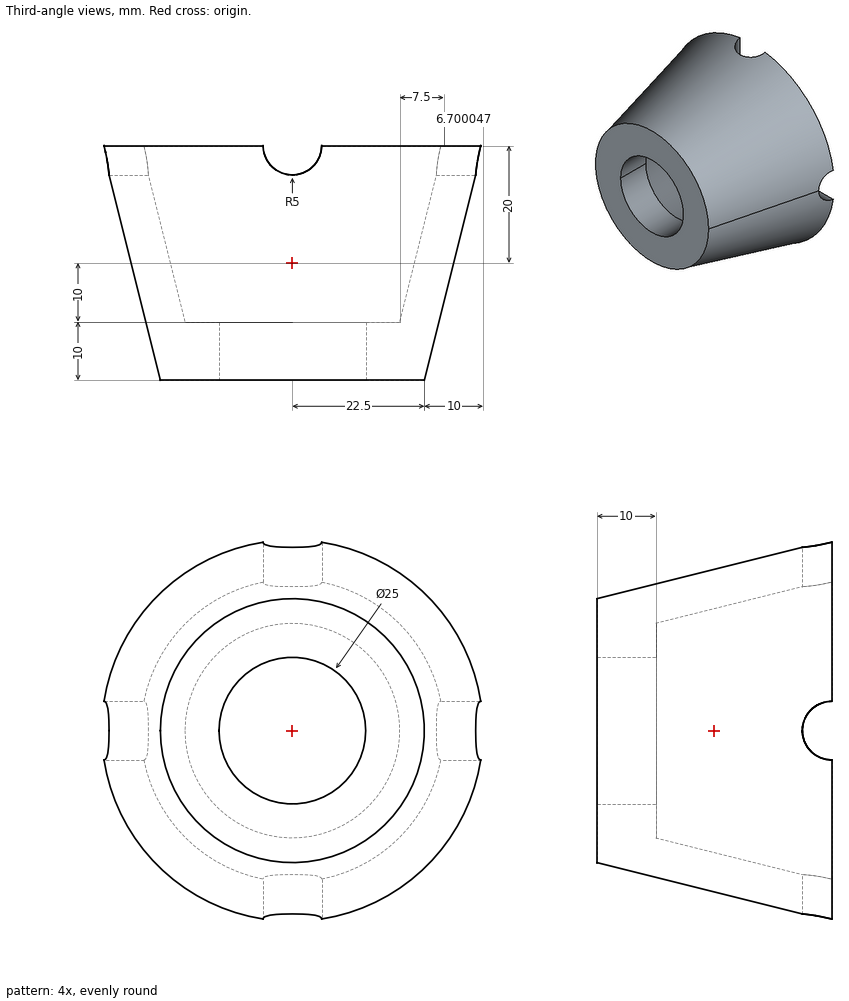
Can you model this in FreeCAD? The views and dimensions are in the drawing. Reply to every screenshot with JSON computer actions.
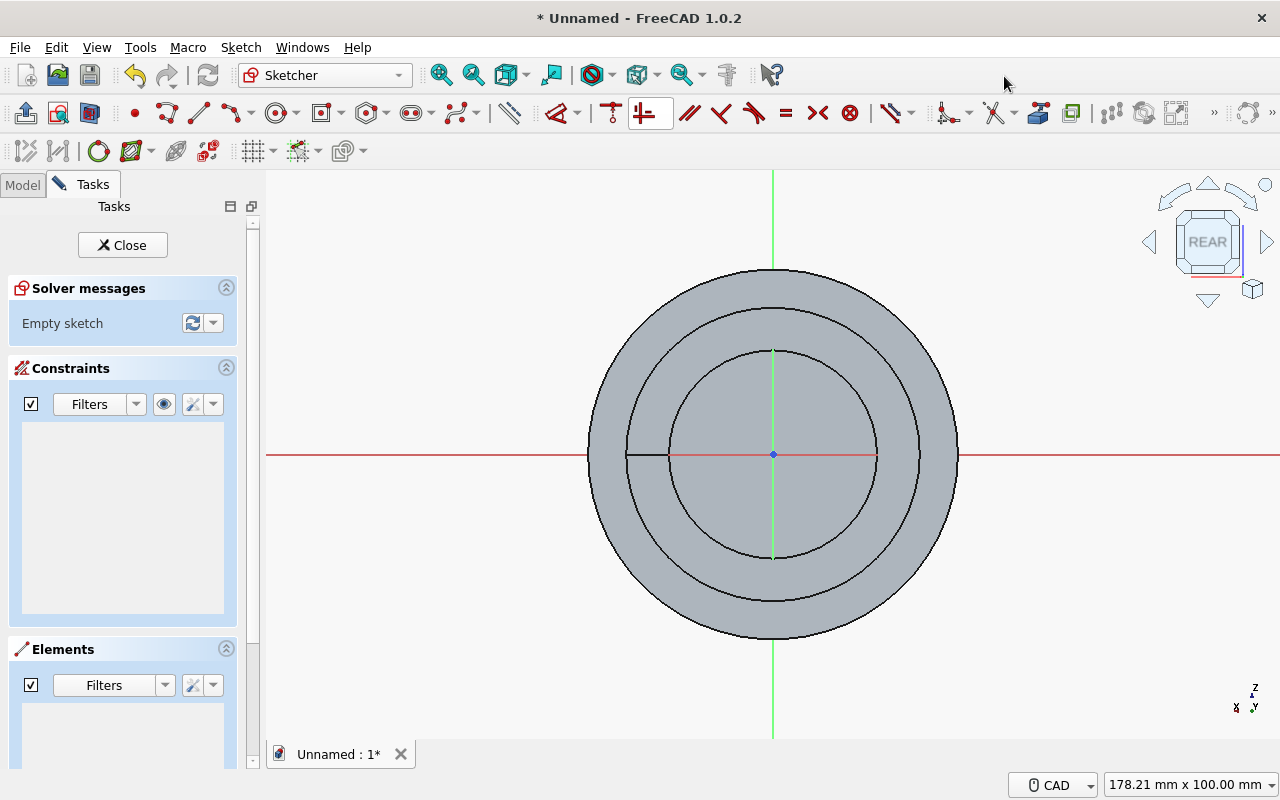
{"action": "scroll", "coordinate": [813, 455], "scroll_direction": "up", "scroll_amount": 5}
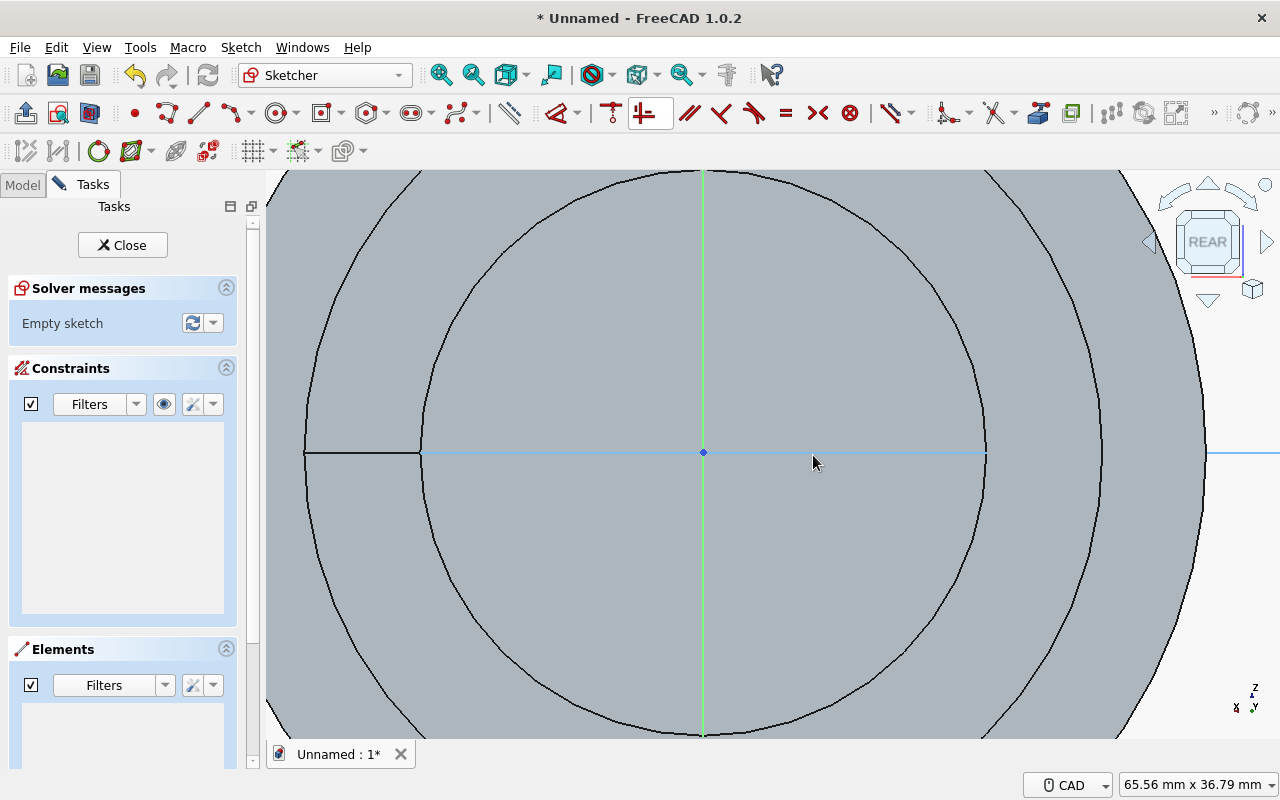
{"action": "left_click", "coordinate": [276, 114]}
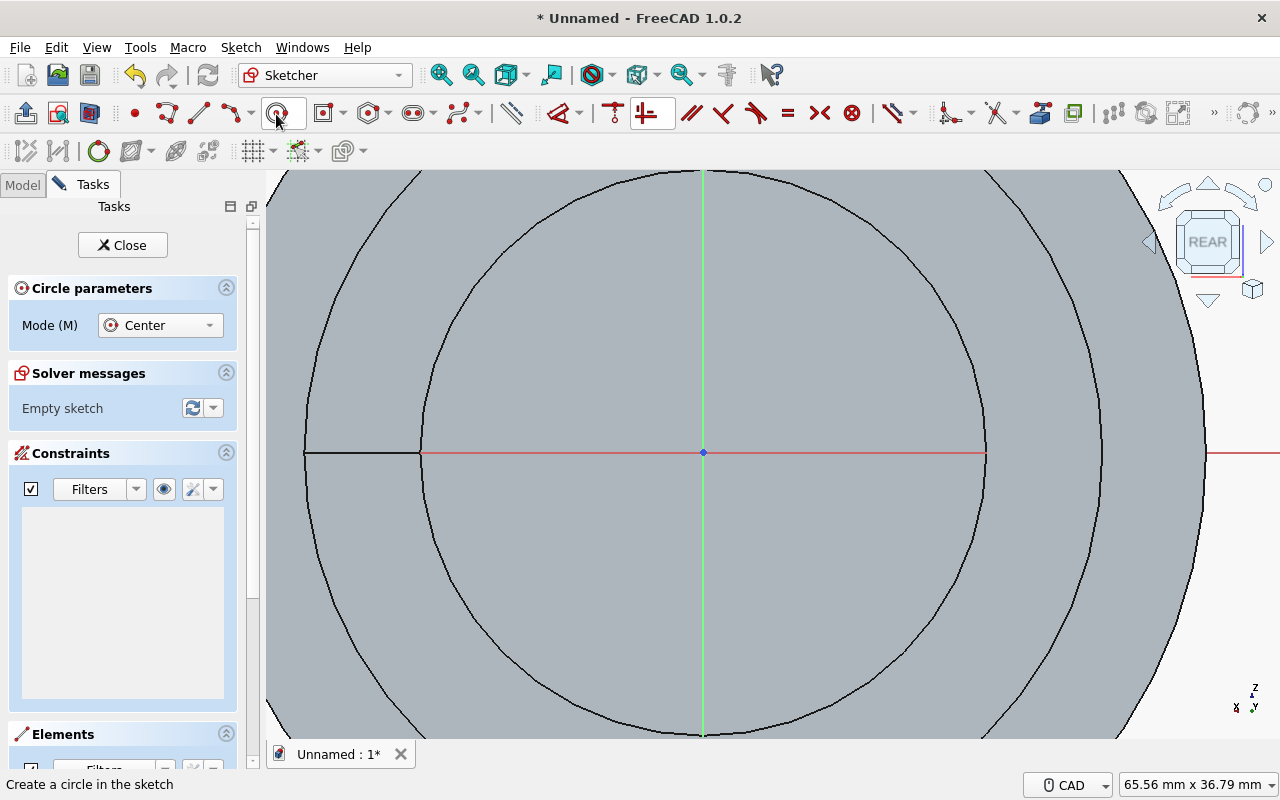
{"action": "left_click", "coordinate": [703, 453]}
{"action": "mouse_move", "coordinate": [840, 316]}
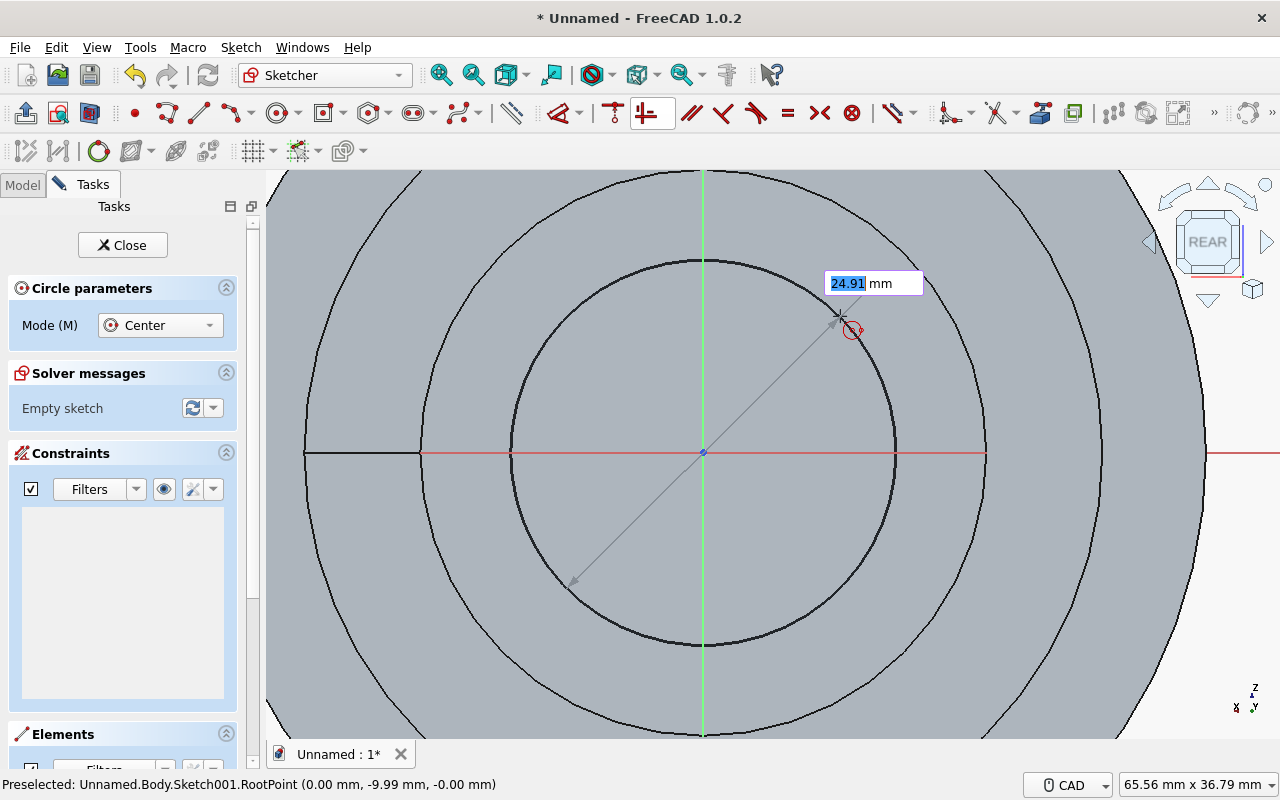
{"action": "type", "text": "25"}
{"action": "key", "text": "Return"}
{"action": "key", "text": "Escape"}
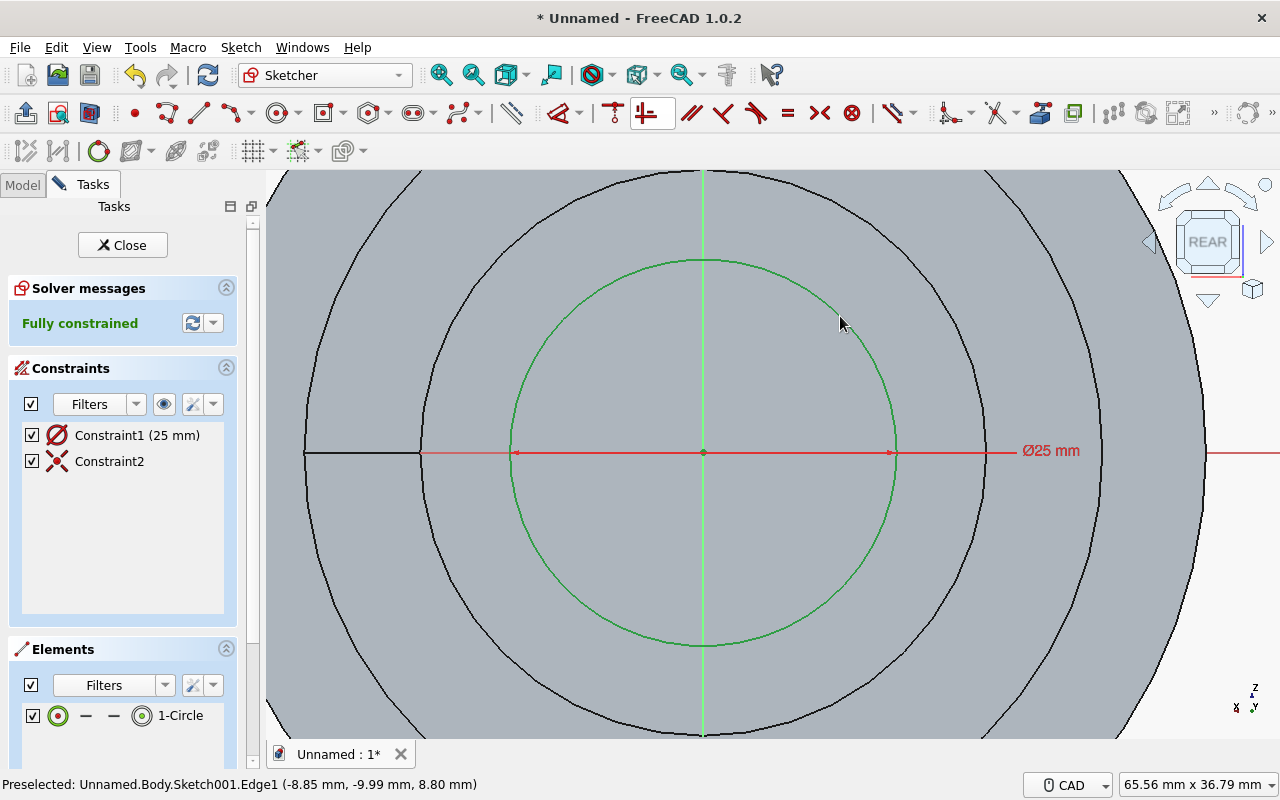
{"action": "left_click", "coordinate": [123, 245]}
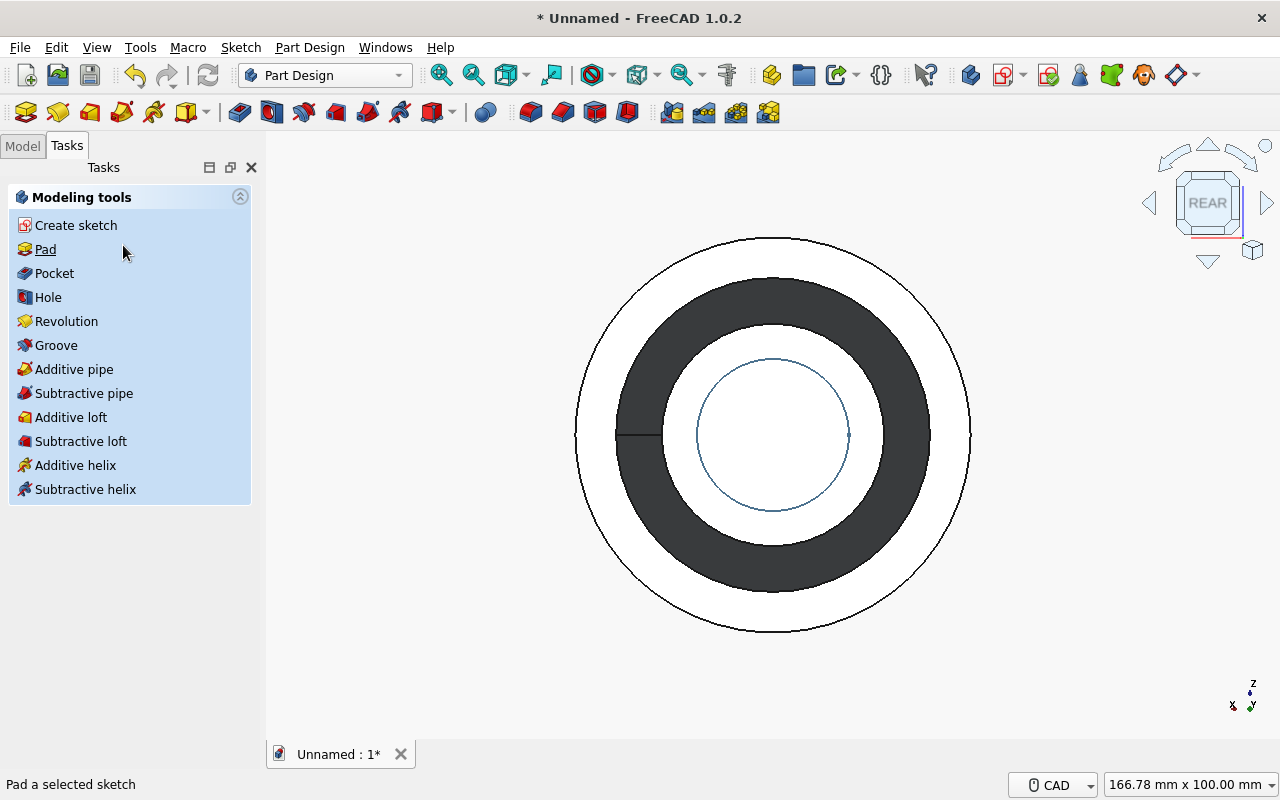
{"action": "left_click", "coordinate": [240, 112]}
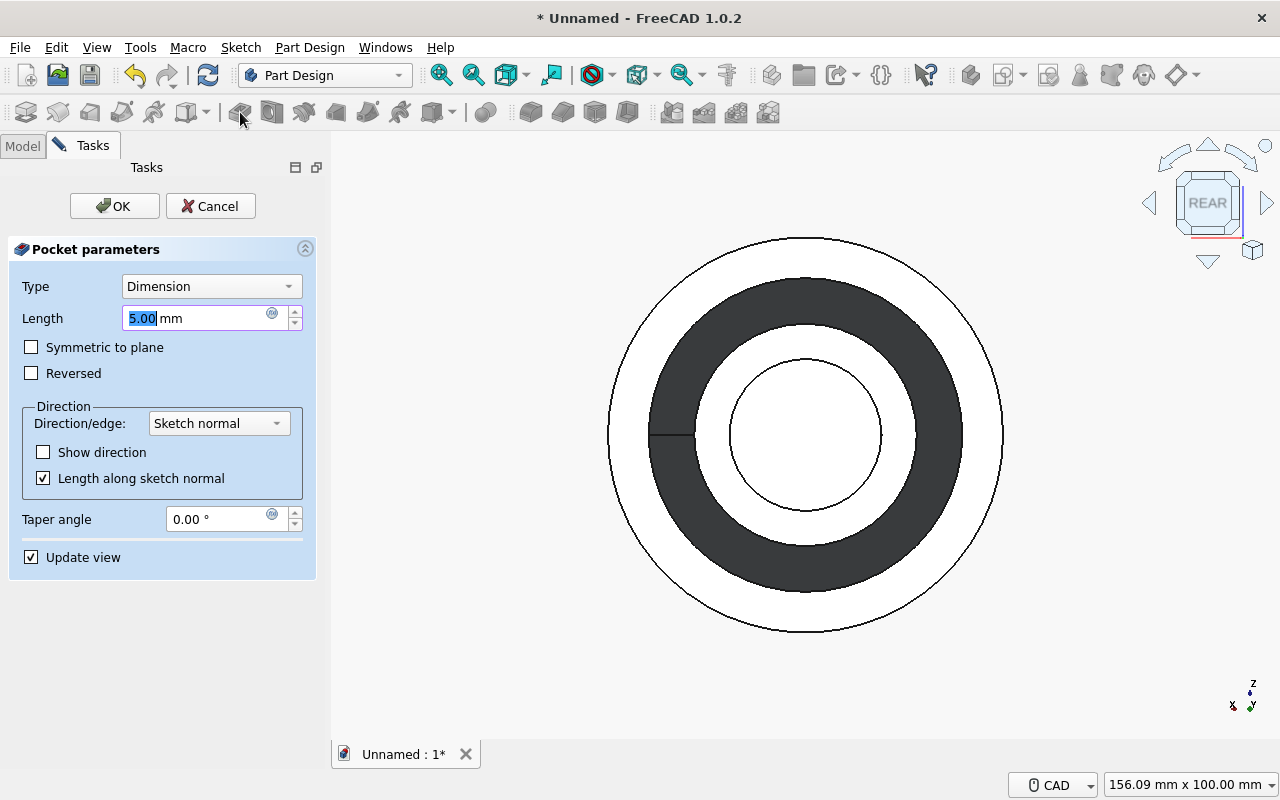
{"action": "type", "text": "10"}
{"action": "key", "text": "Tab"}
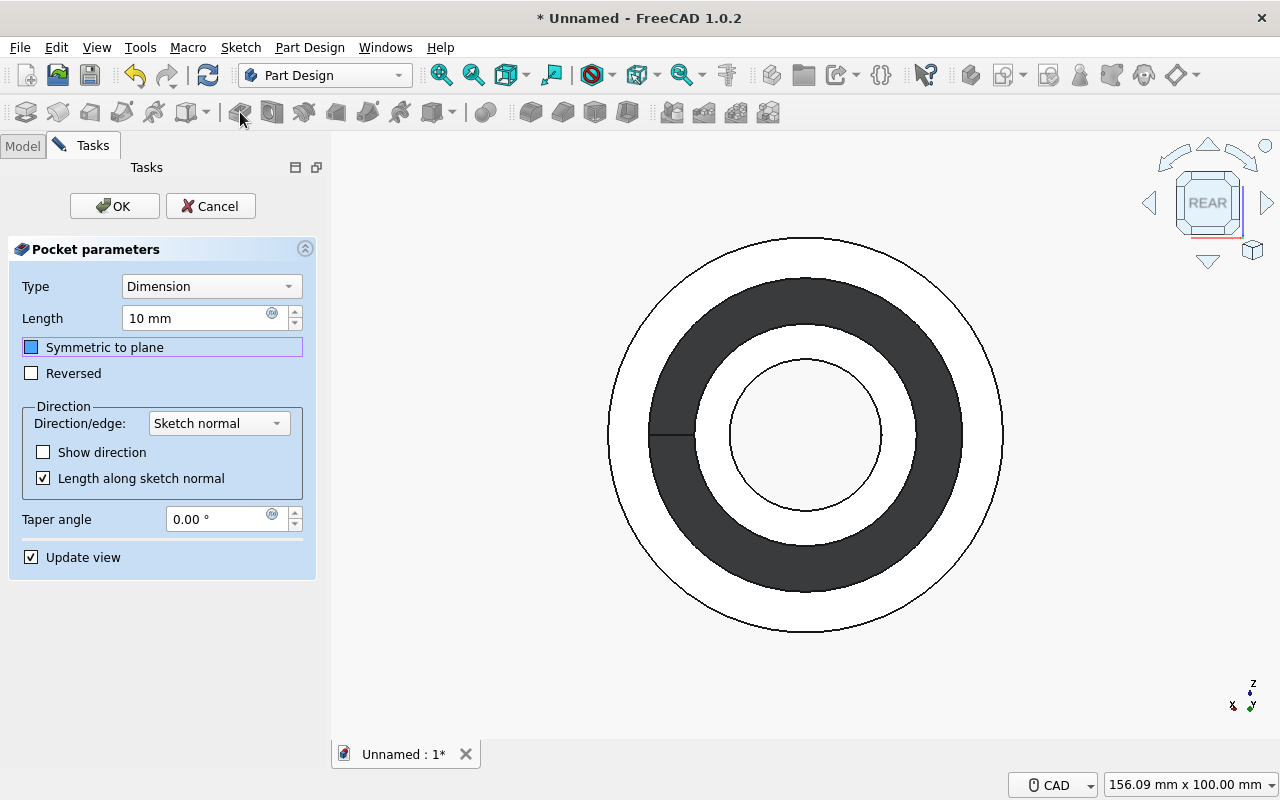
{"action": "left_click", "coordinate": [115, 206]}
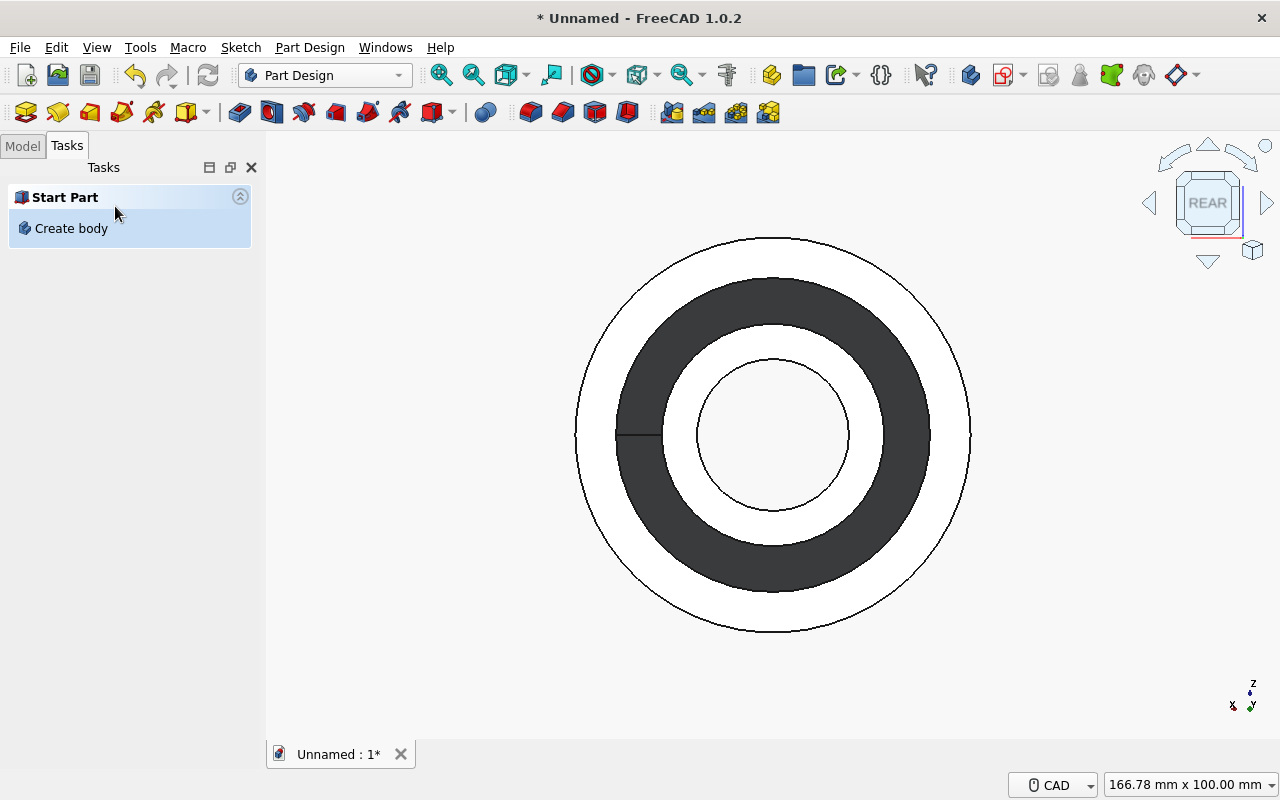
{"action": "left_click", "coordinate": [1004, 76]}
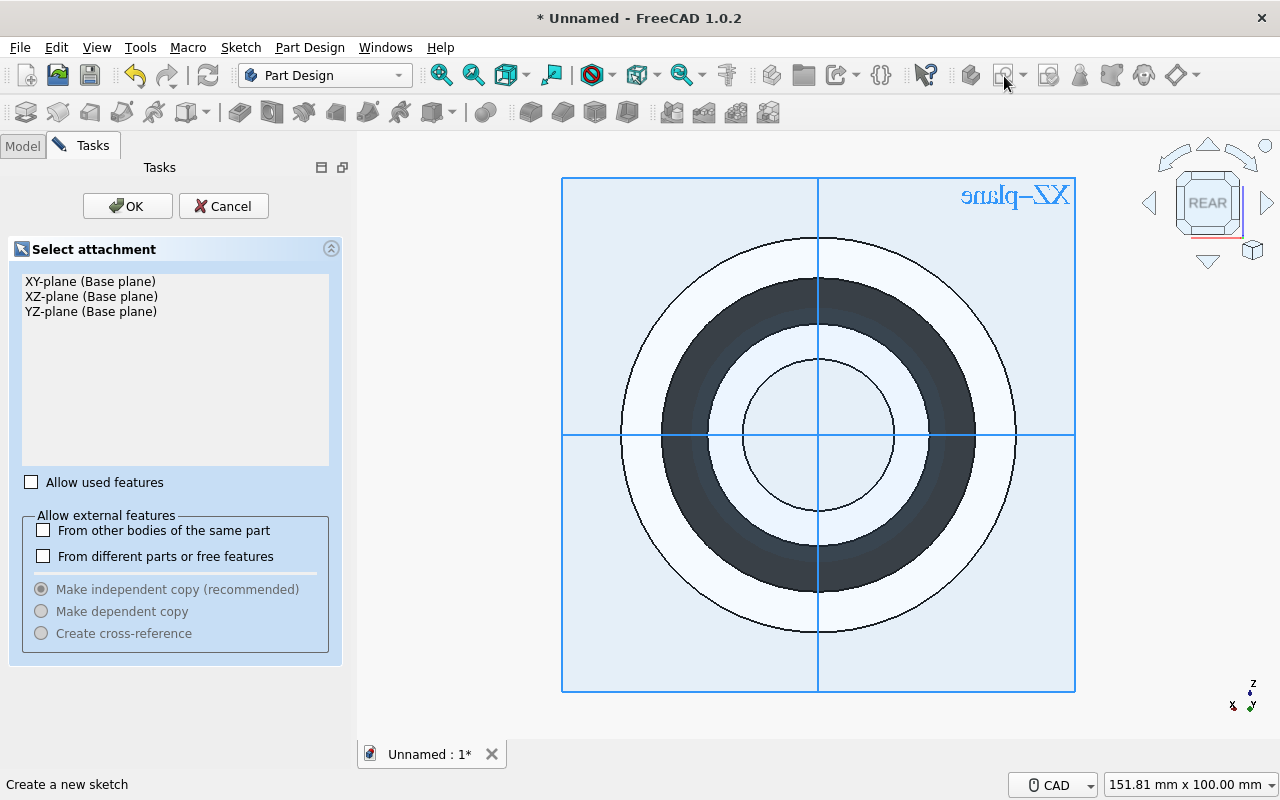
{"action": "left_click", "coordinate": [82, 282]}